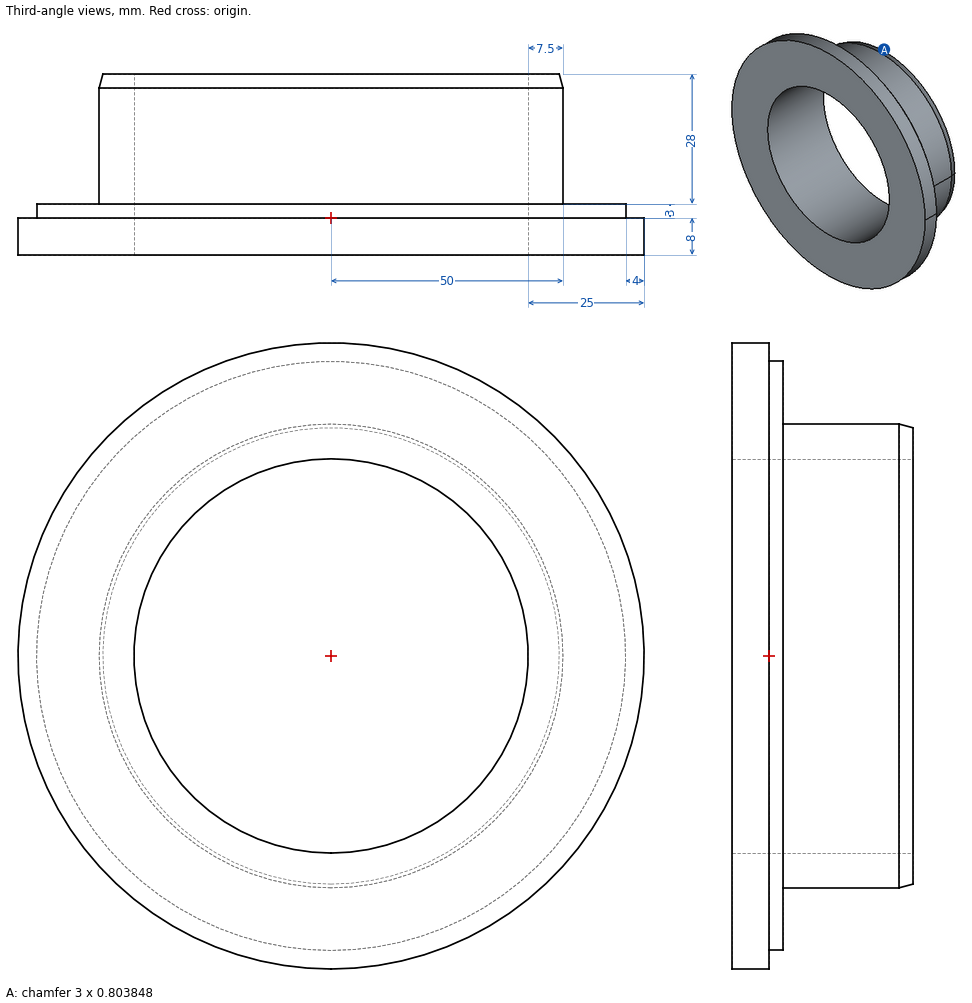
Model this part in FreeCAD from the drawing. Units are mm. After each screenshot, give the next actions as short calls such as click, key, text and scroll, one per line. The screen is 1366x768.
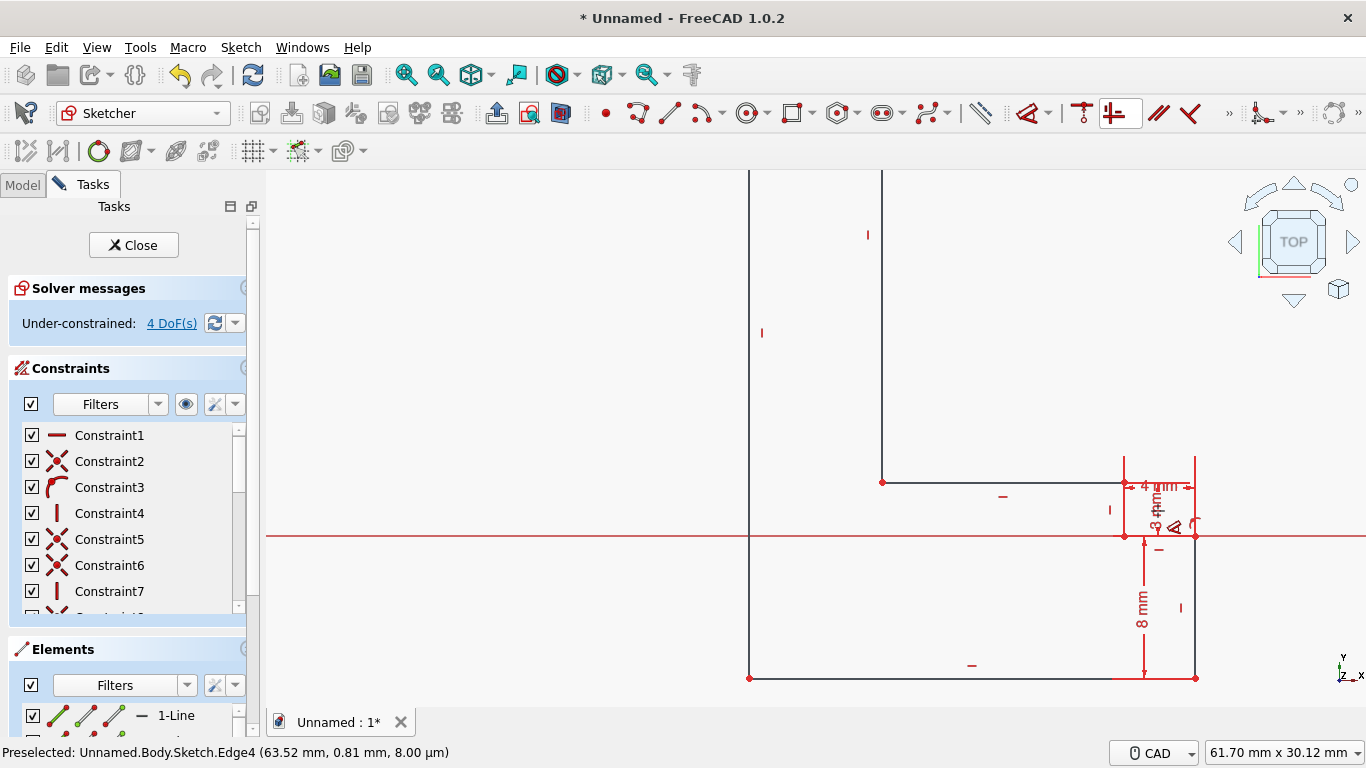
click(883, 679)
click(972, 645)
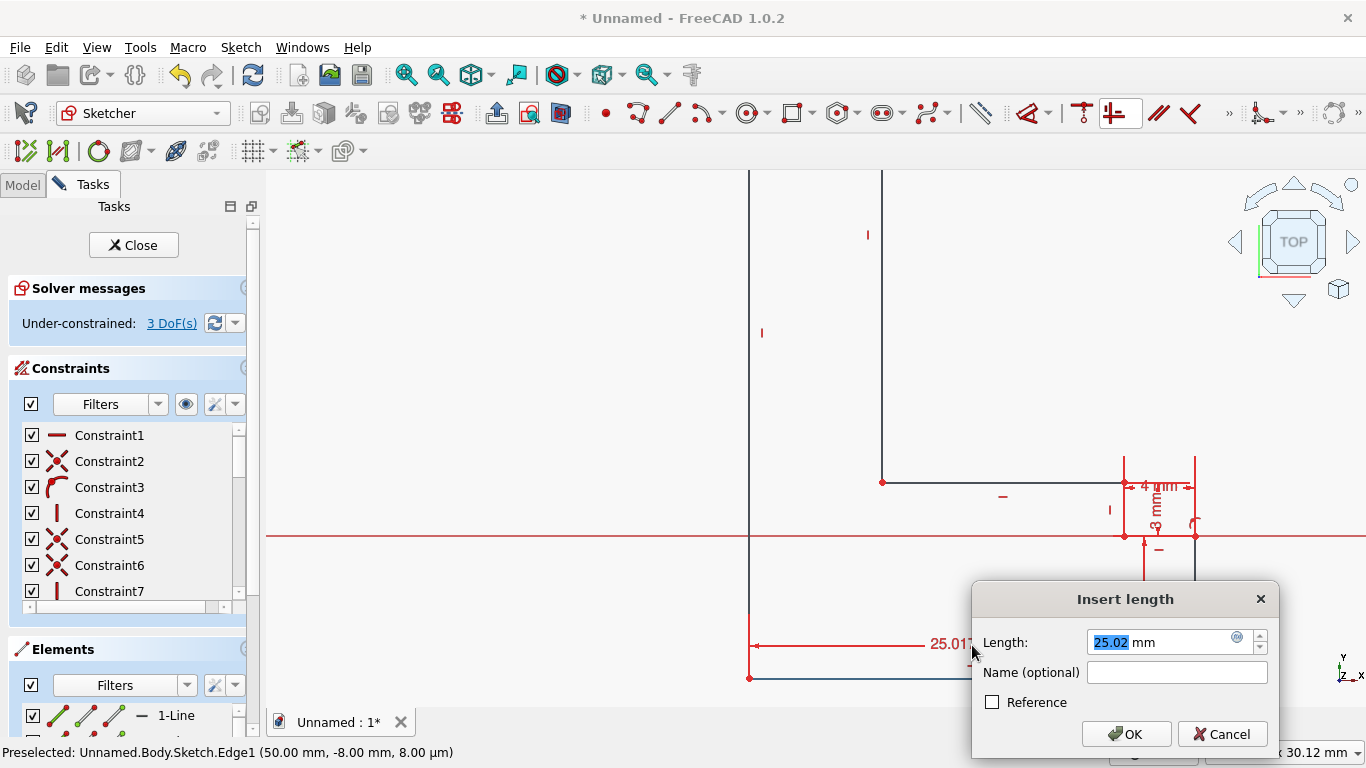
text(25)
key(Return)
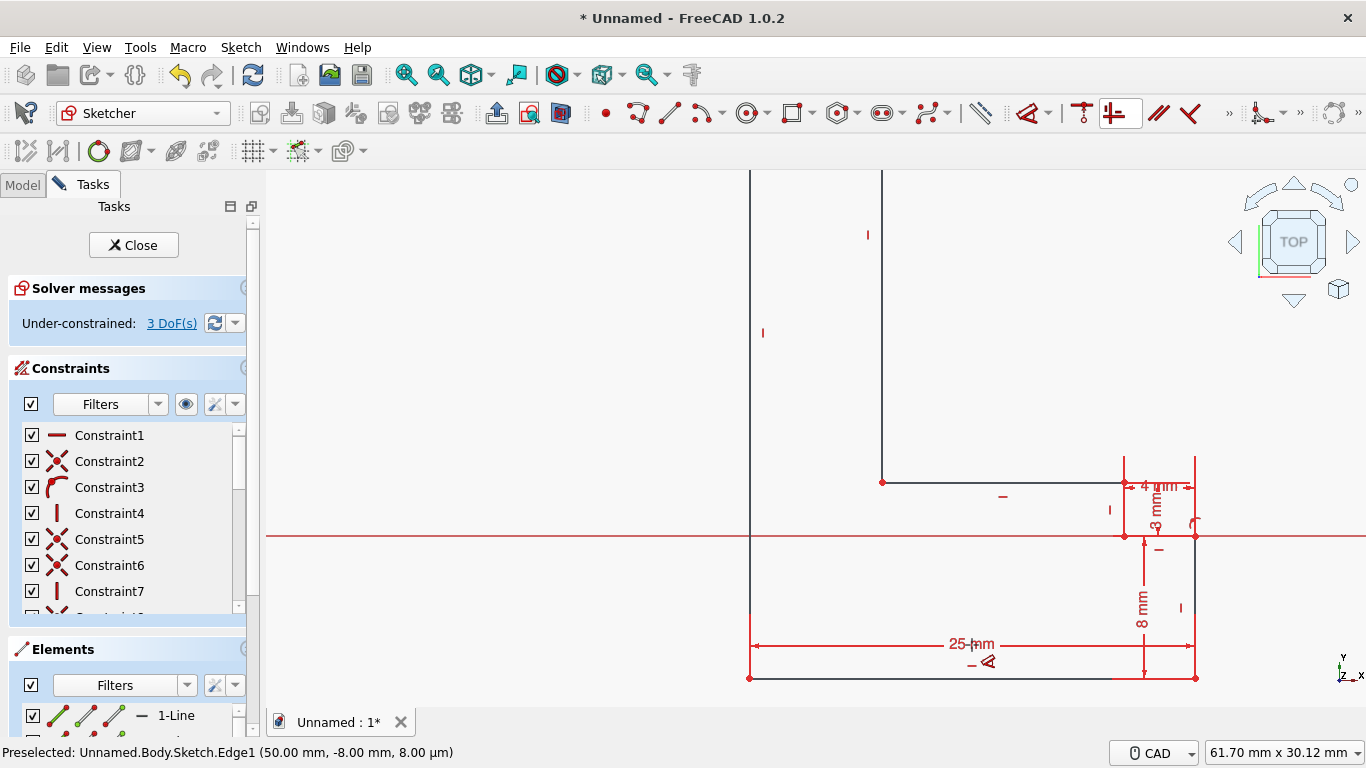
click(882, 334)
click(916, 340)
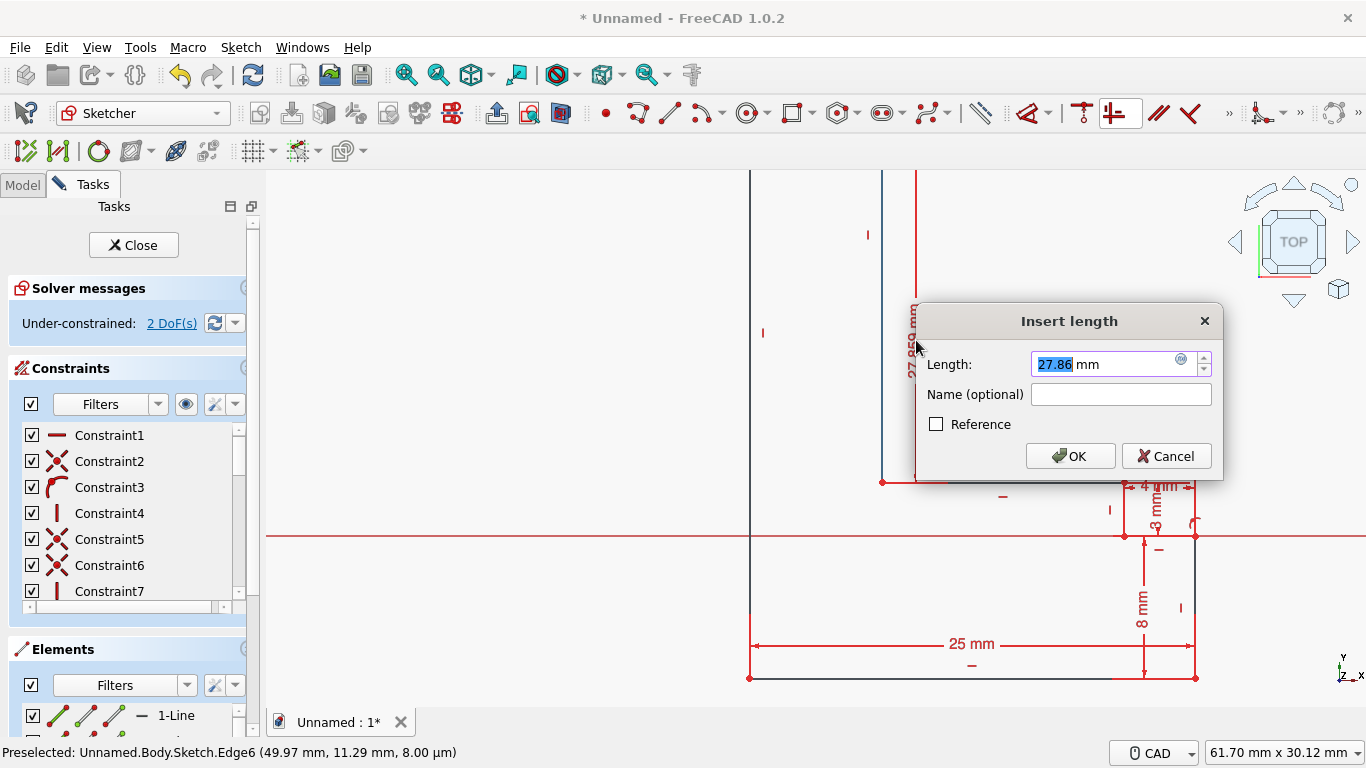
text(28)
key(Return)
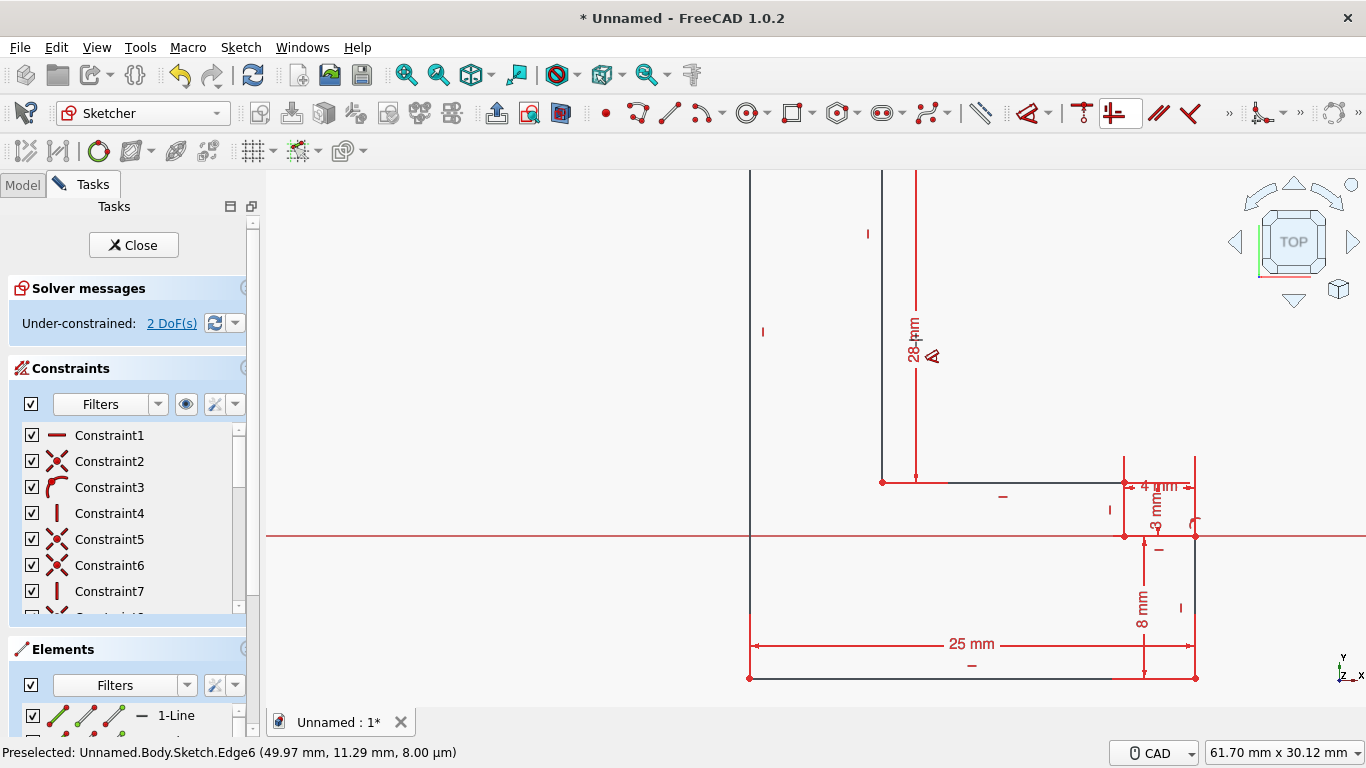
scroll(873, 526, down, 4)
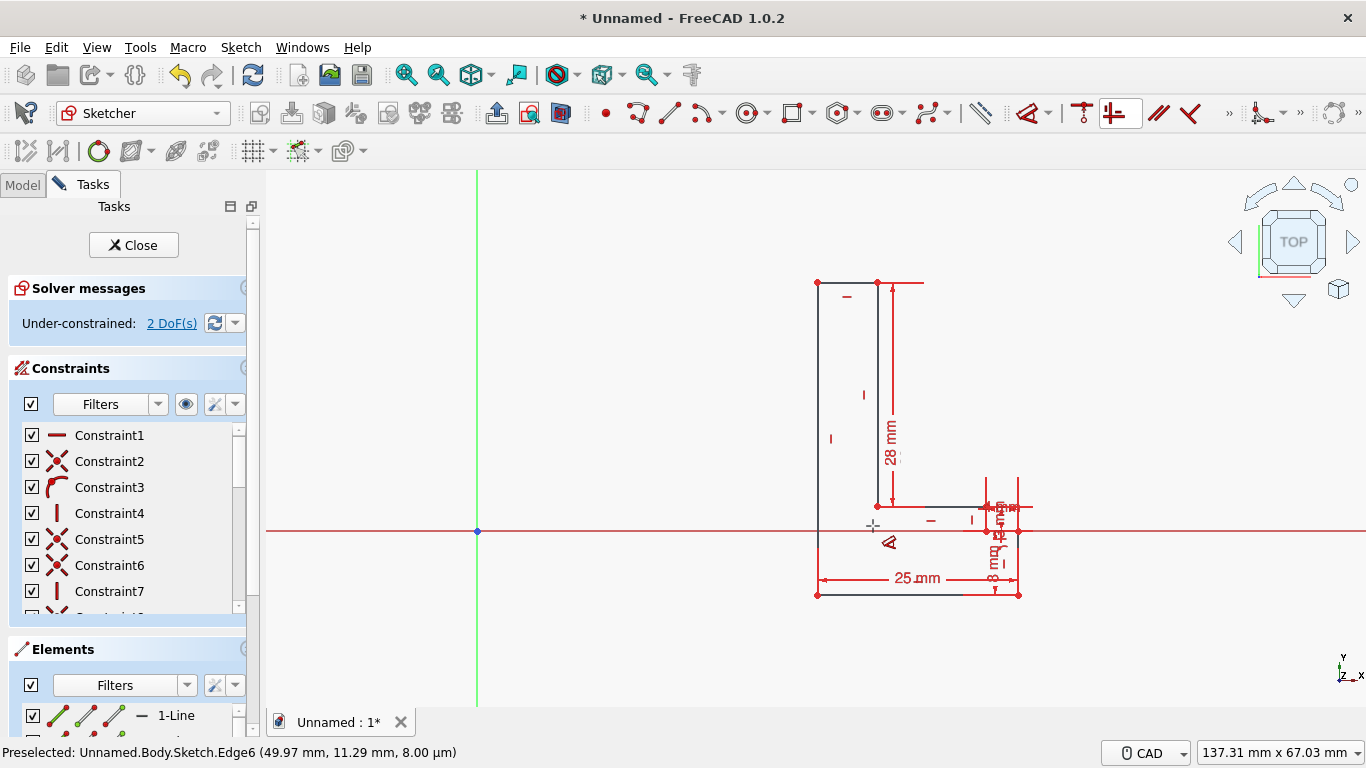
click(860, 283)
click(848, 249)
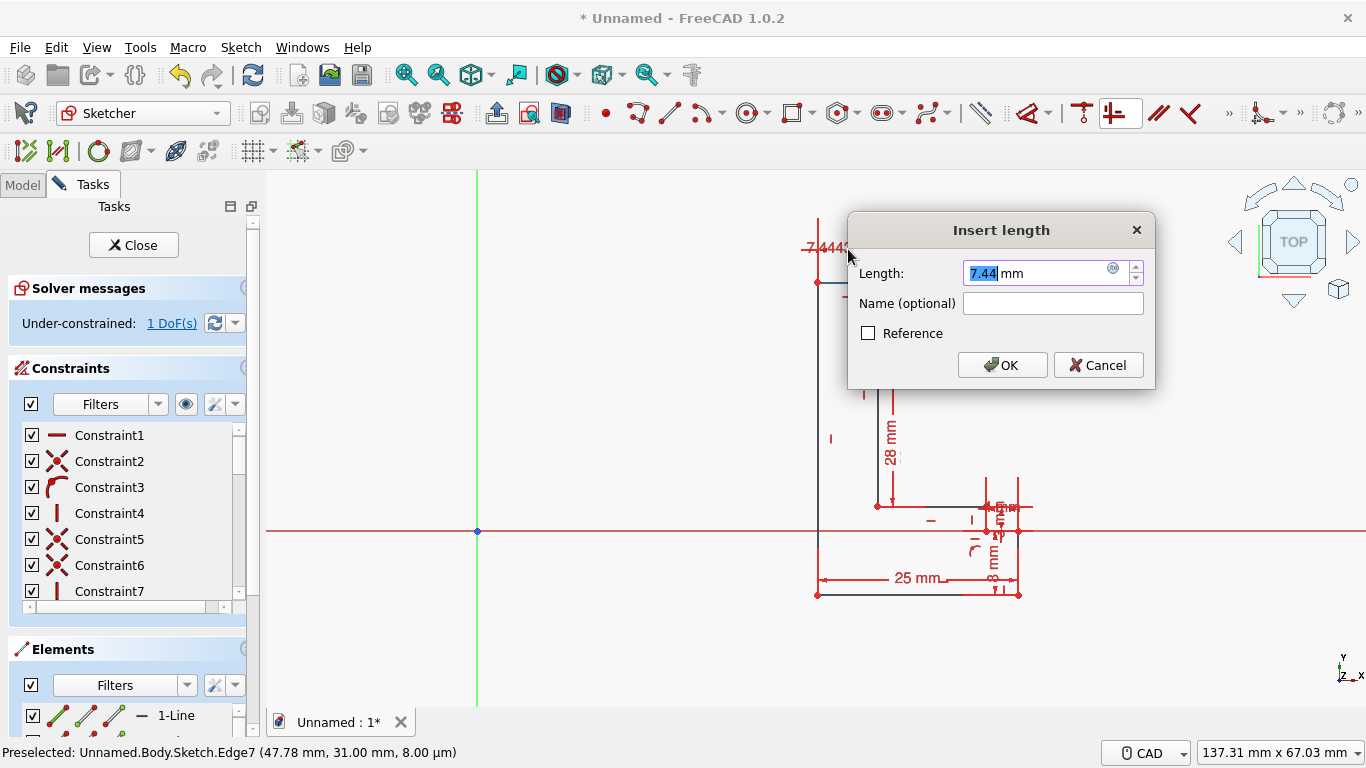
text(7.5)
key(Return)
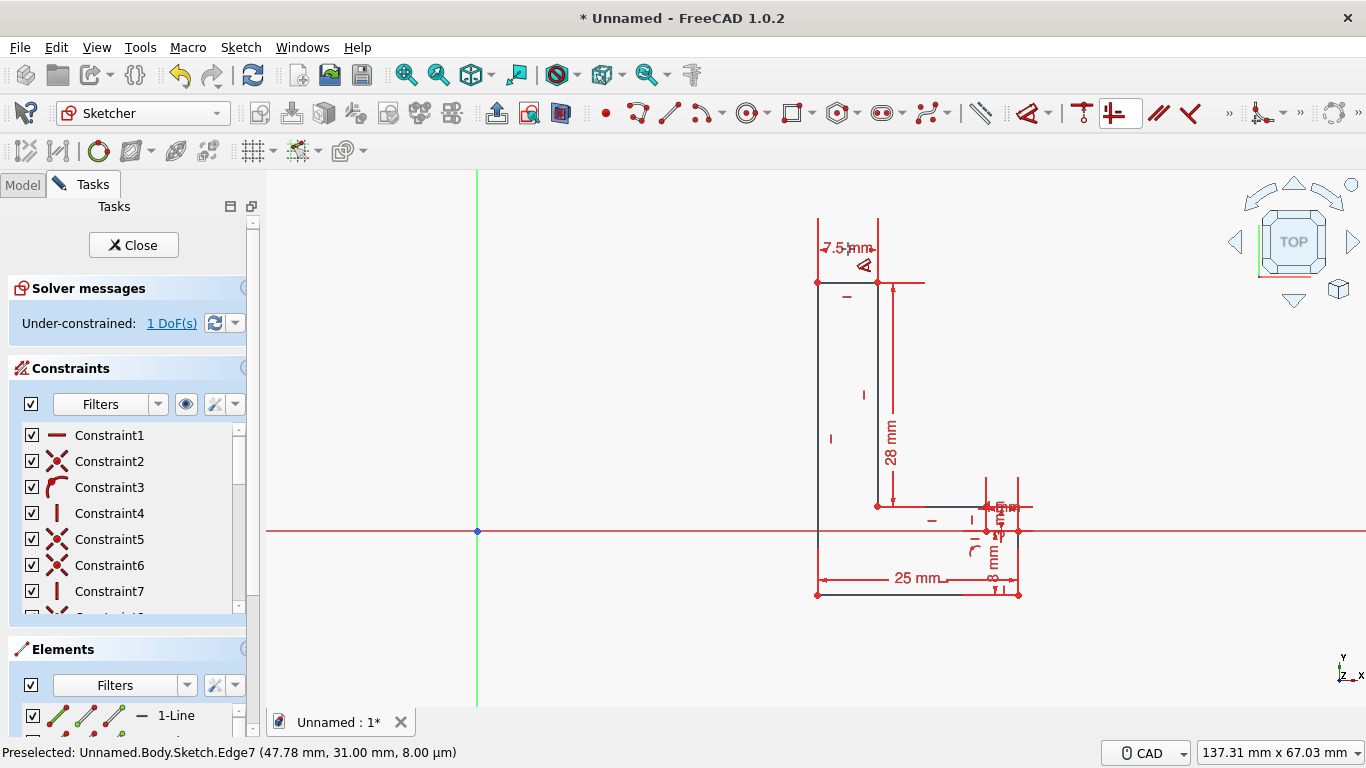
click(878, 507)
click(678, 565)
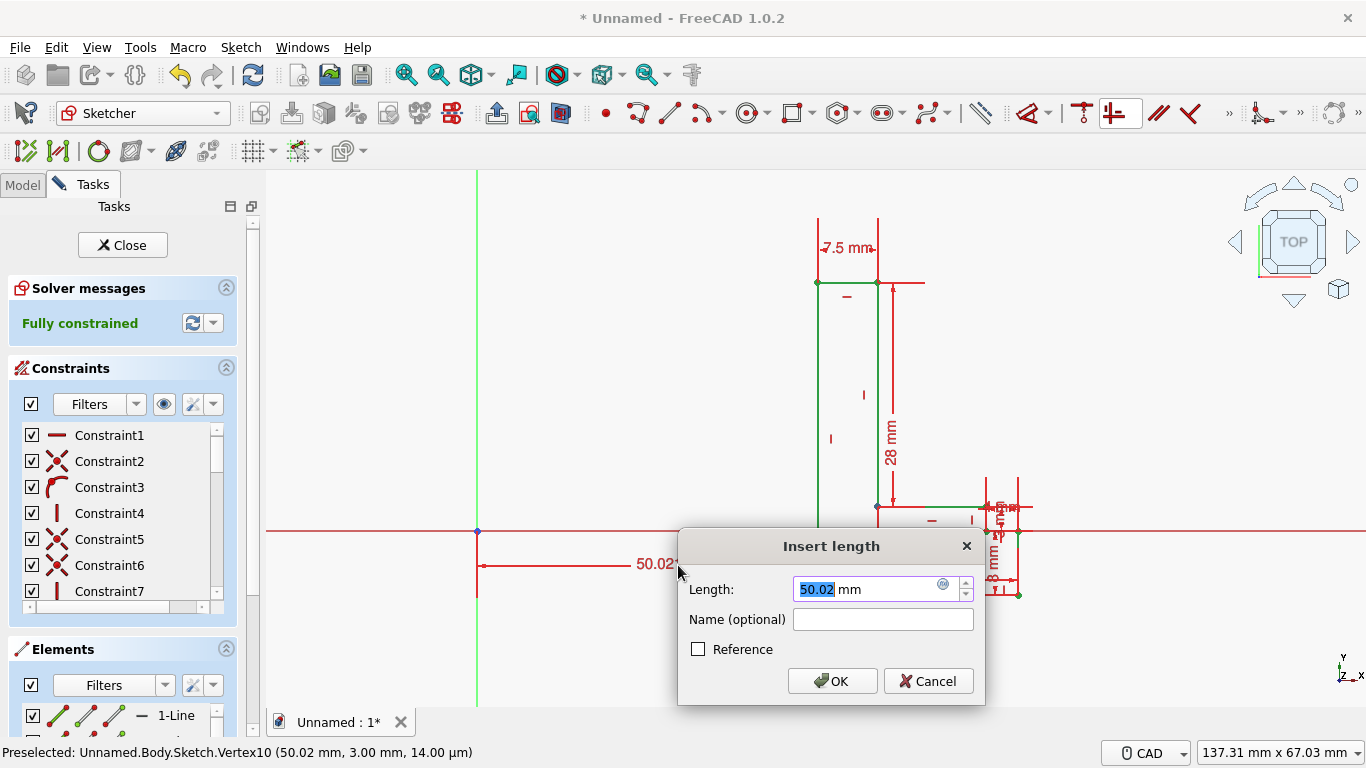
text(50)
key(Return)
key(Escape)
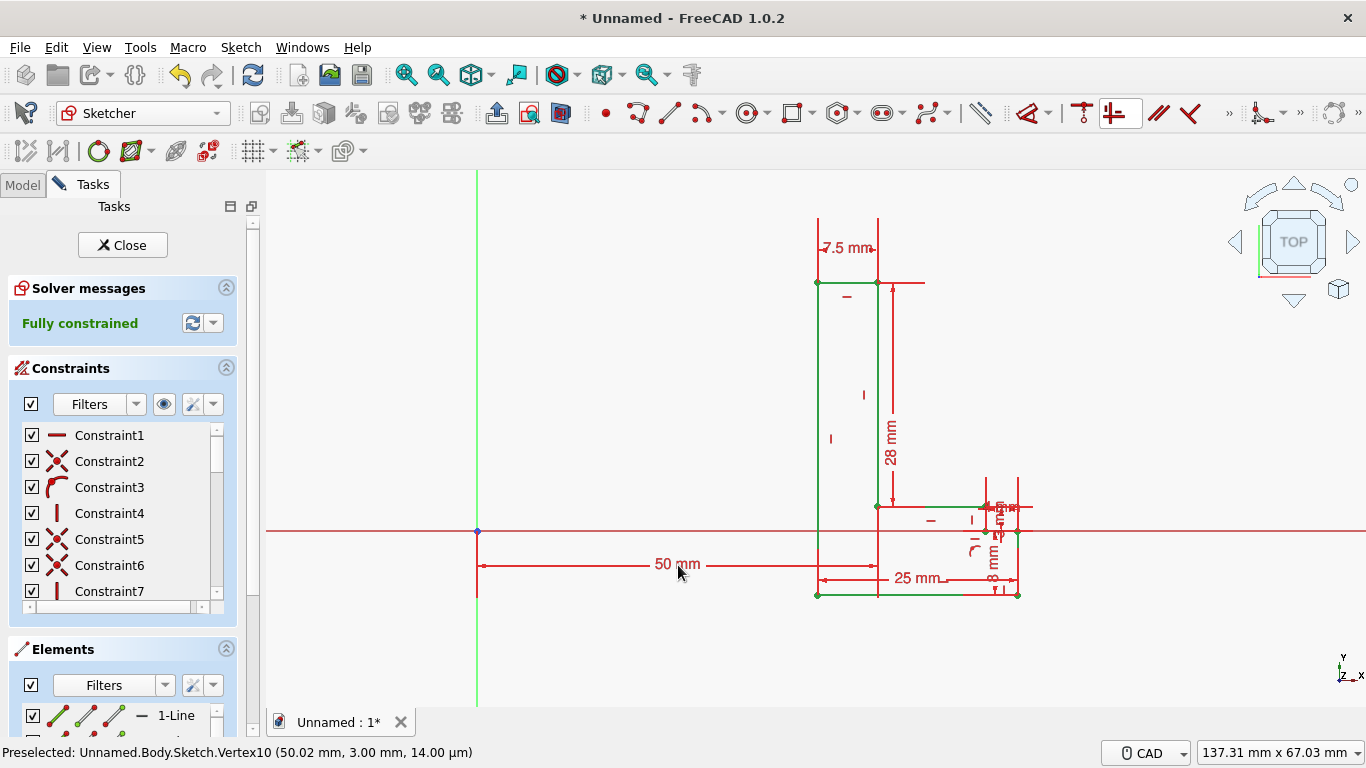
click(123, 245)